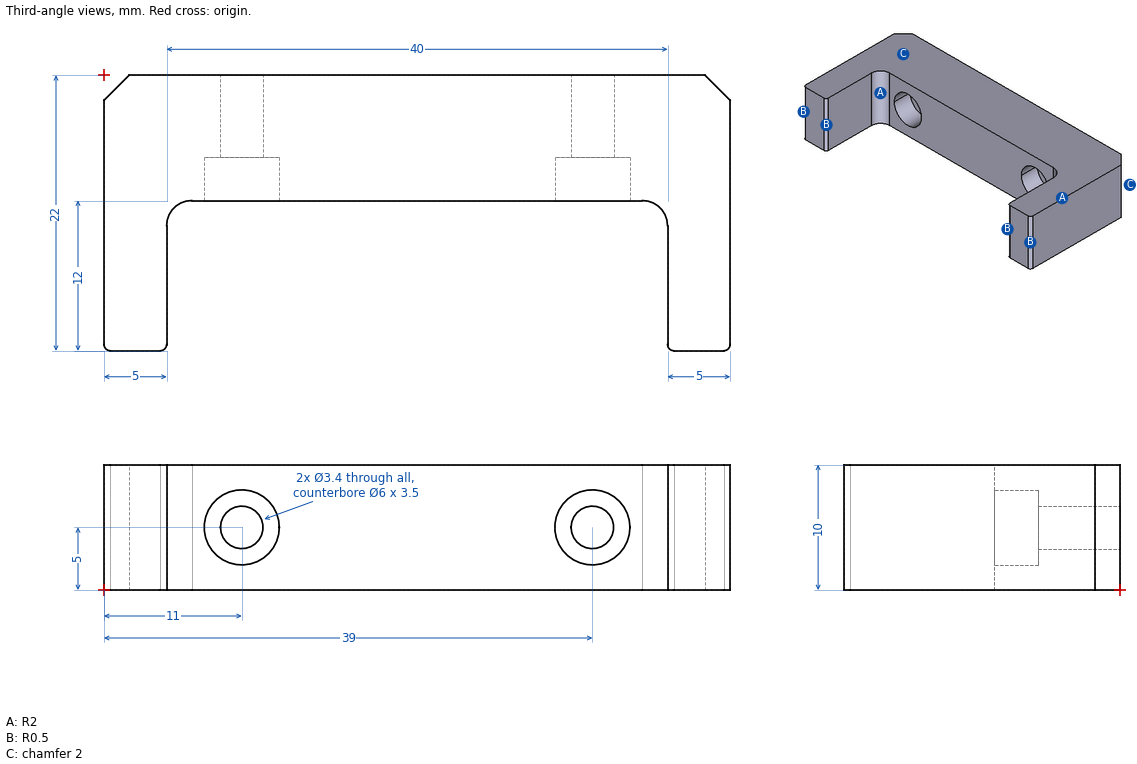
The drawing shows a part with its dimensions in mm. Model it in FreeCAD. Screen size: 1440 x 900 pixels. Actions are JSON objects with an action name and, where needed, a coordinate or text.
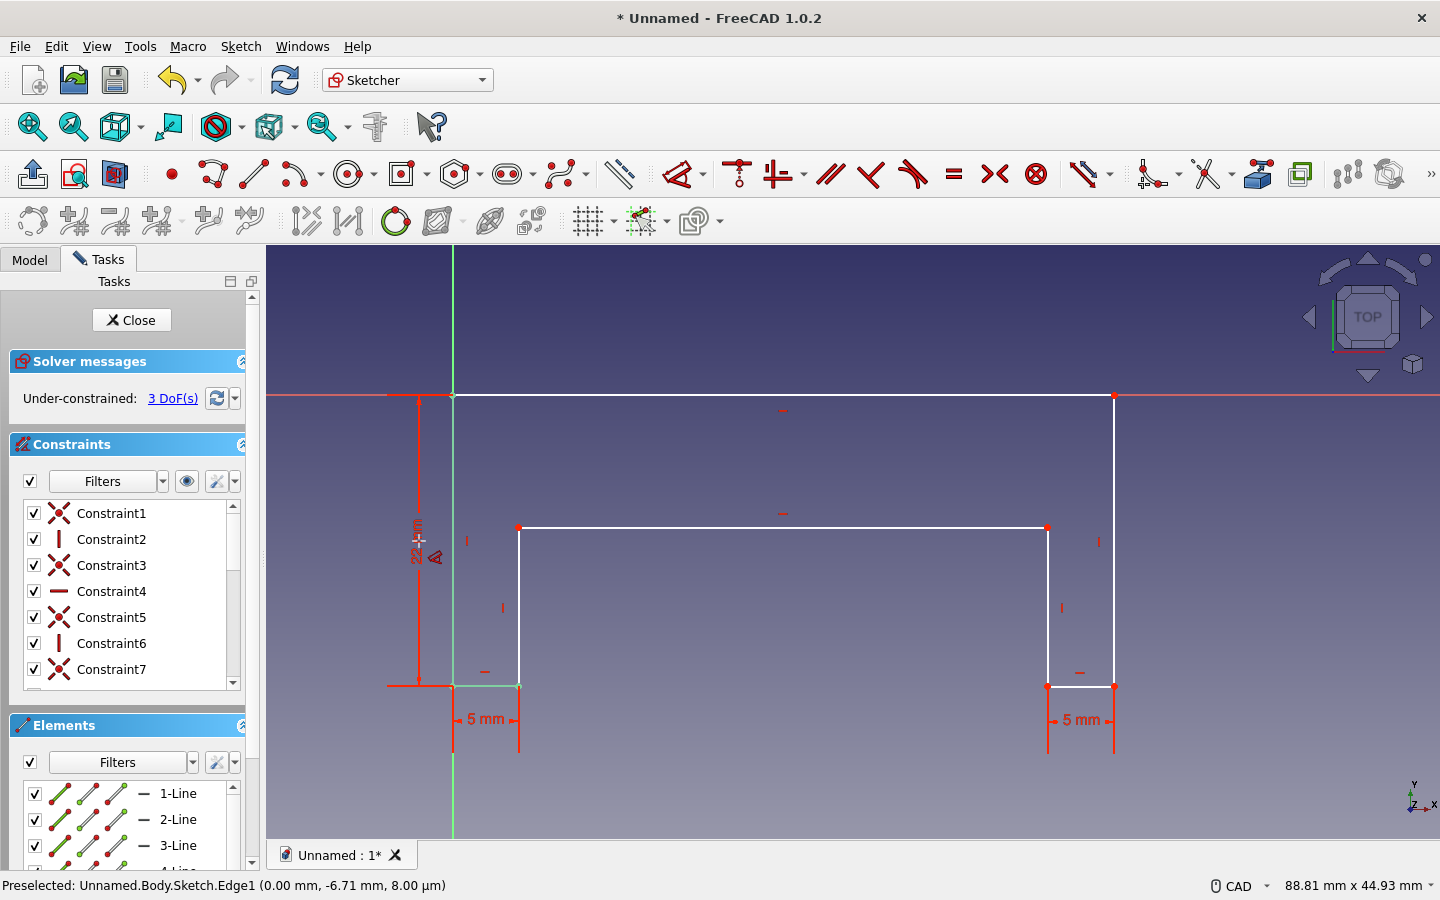
{"action": "left_click", "coordinate": [519, 639]}
{"action": "left_click", "coordinate": [485, 607]}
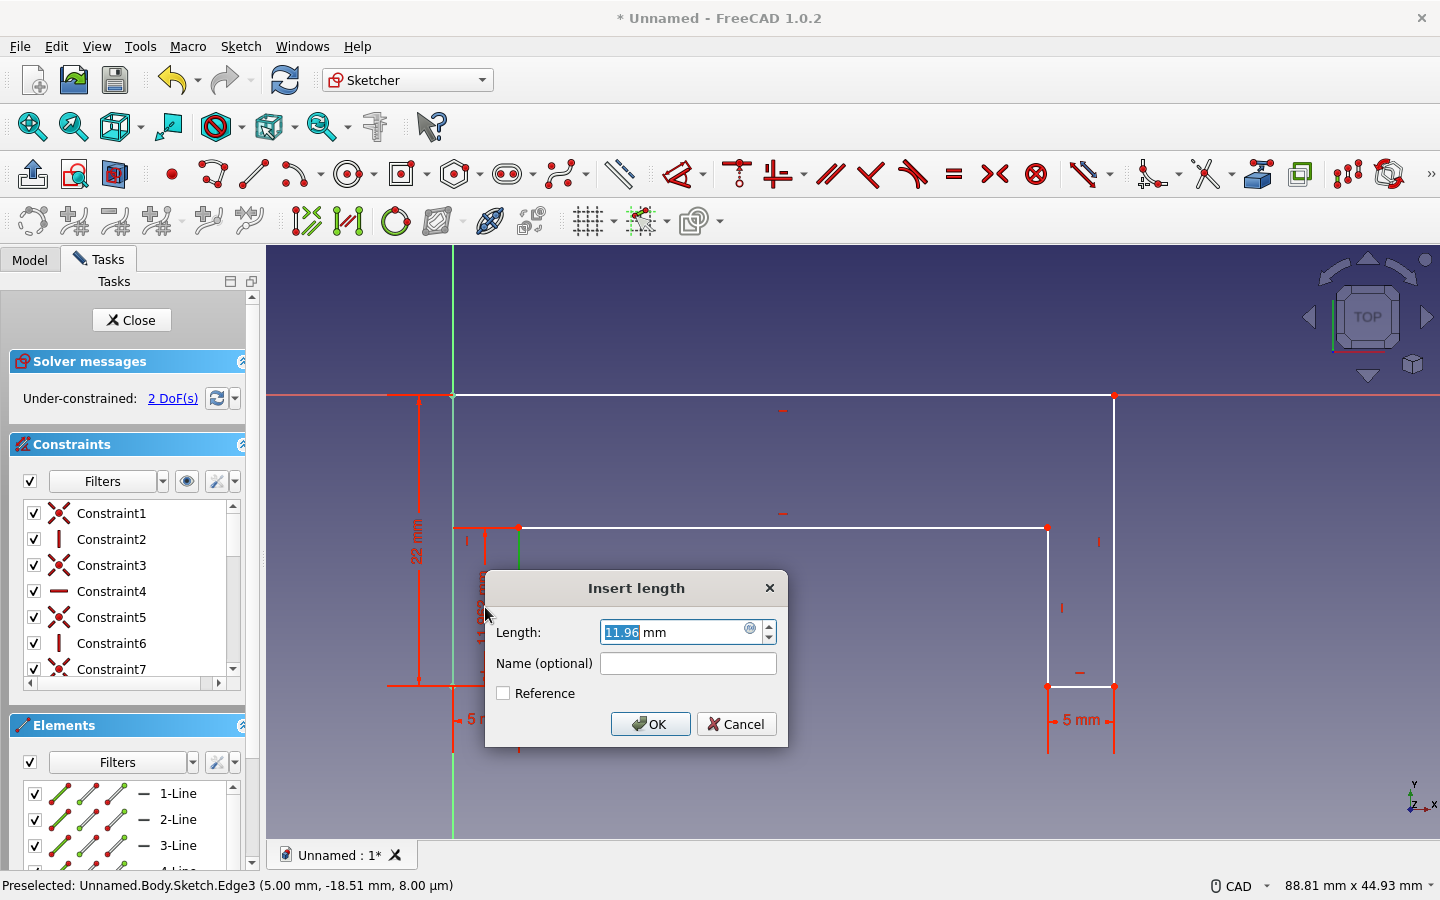
{"action": "type", "text": "12"}
{"action": "key", "text": "Return"}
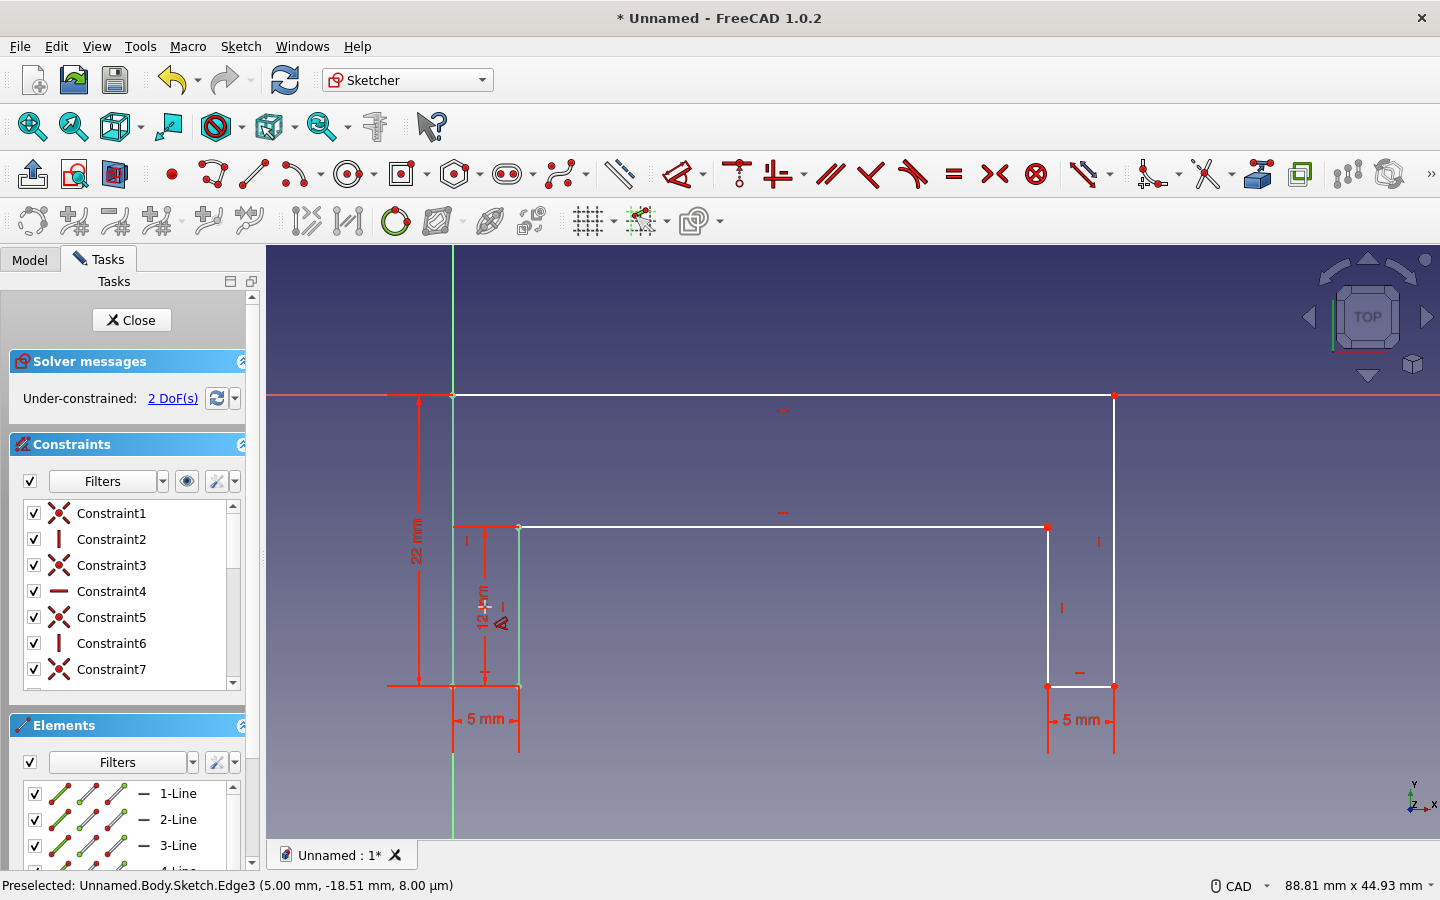
{"action": "left_click", "coordinate": [677, 527]}
{"action": "left_click", "coordinate": [783, 493]}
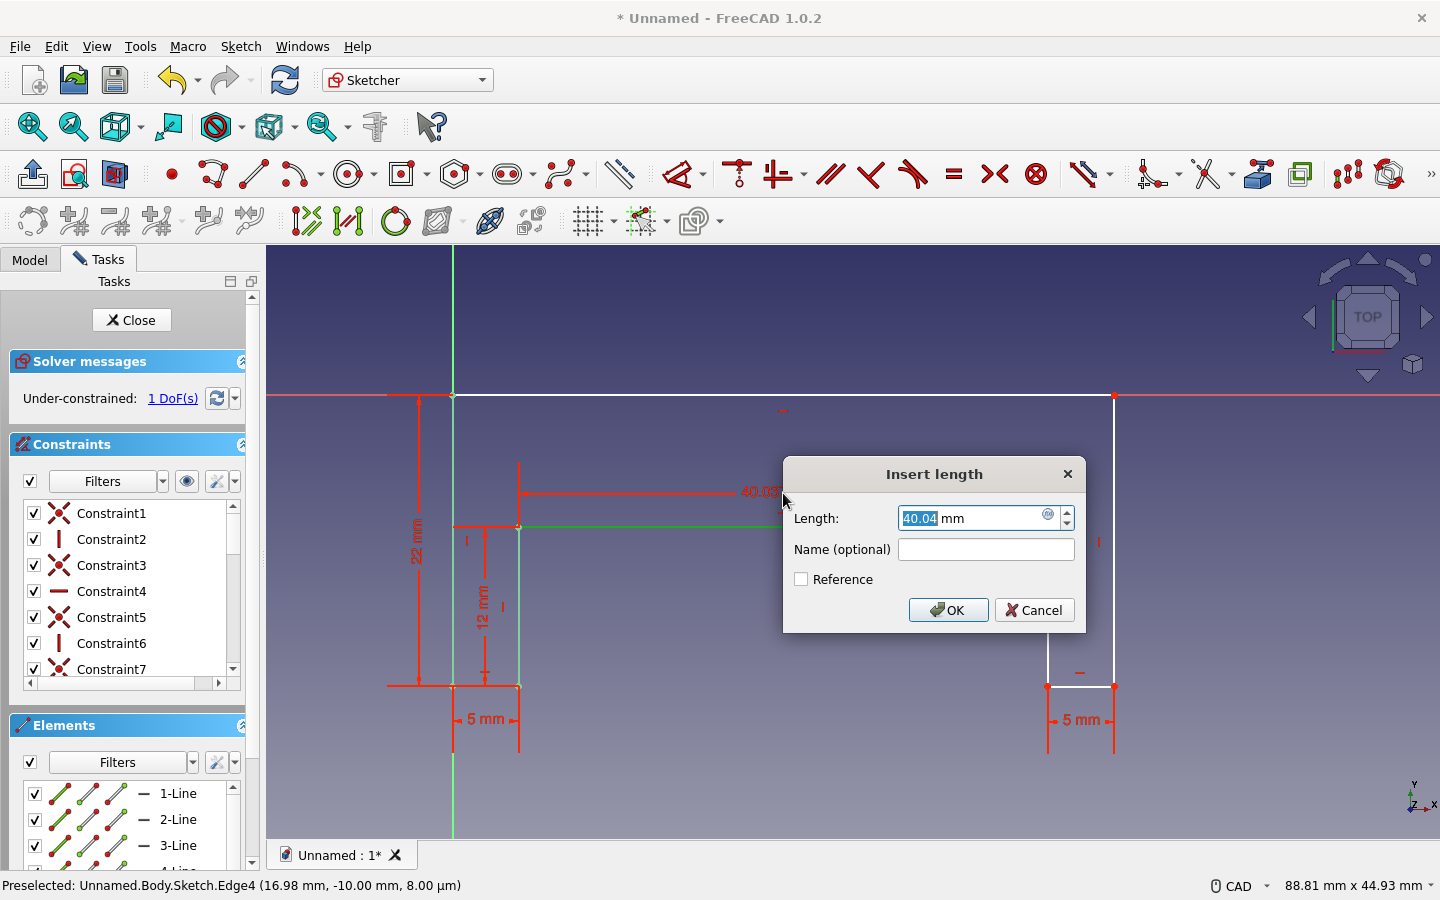
{"action": "type", "text": "40"}
{"action": "key", "text": "Return"}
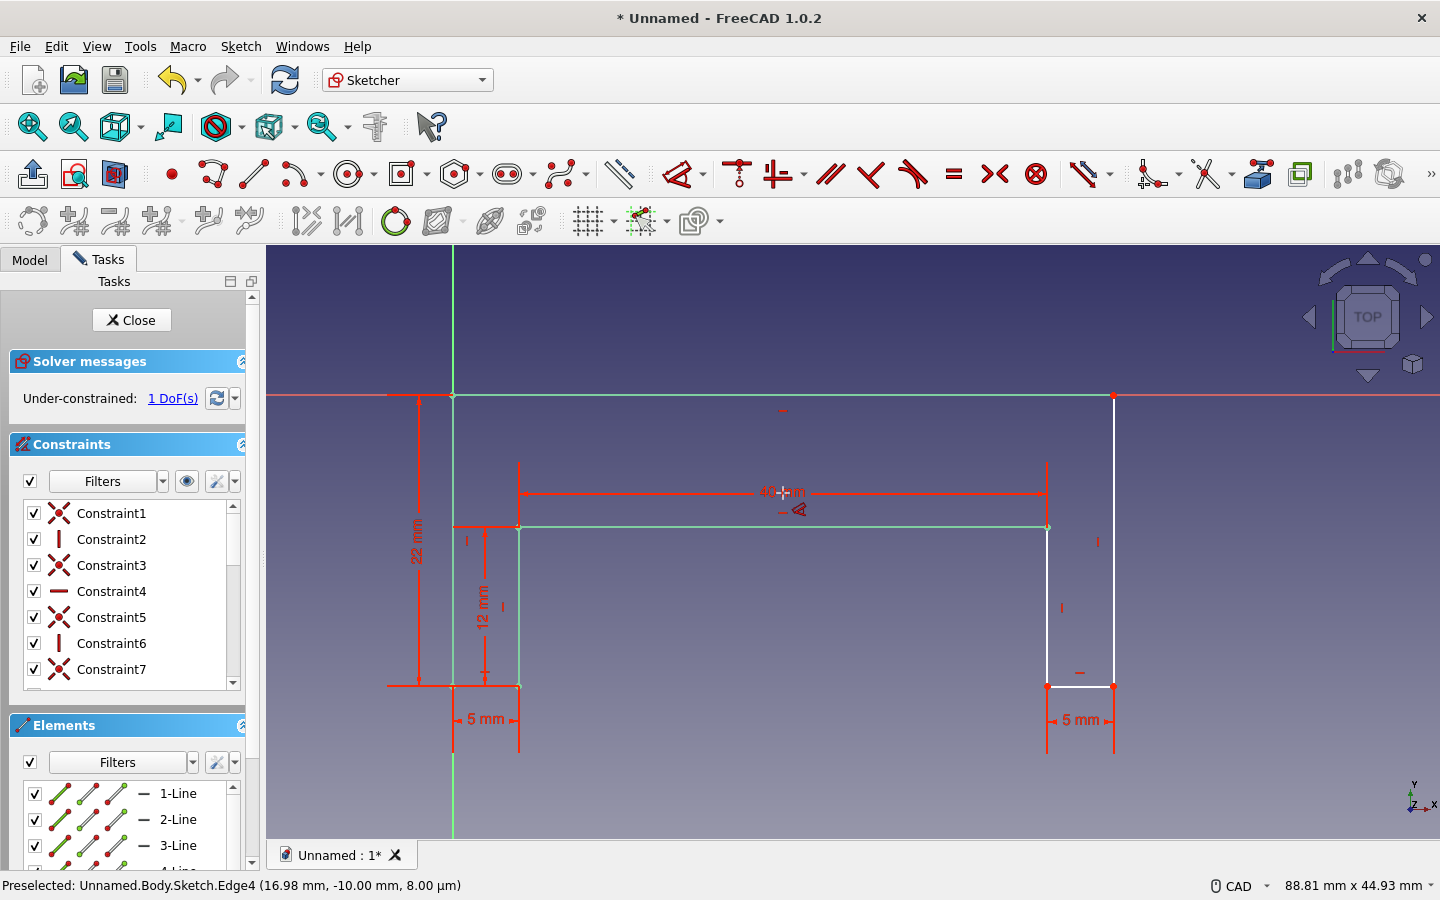
{"action": "left_click", "coordinate": [1047, 575]}
{"action": "left_click", "coordinate": [1081, 607]}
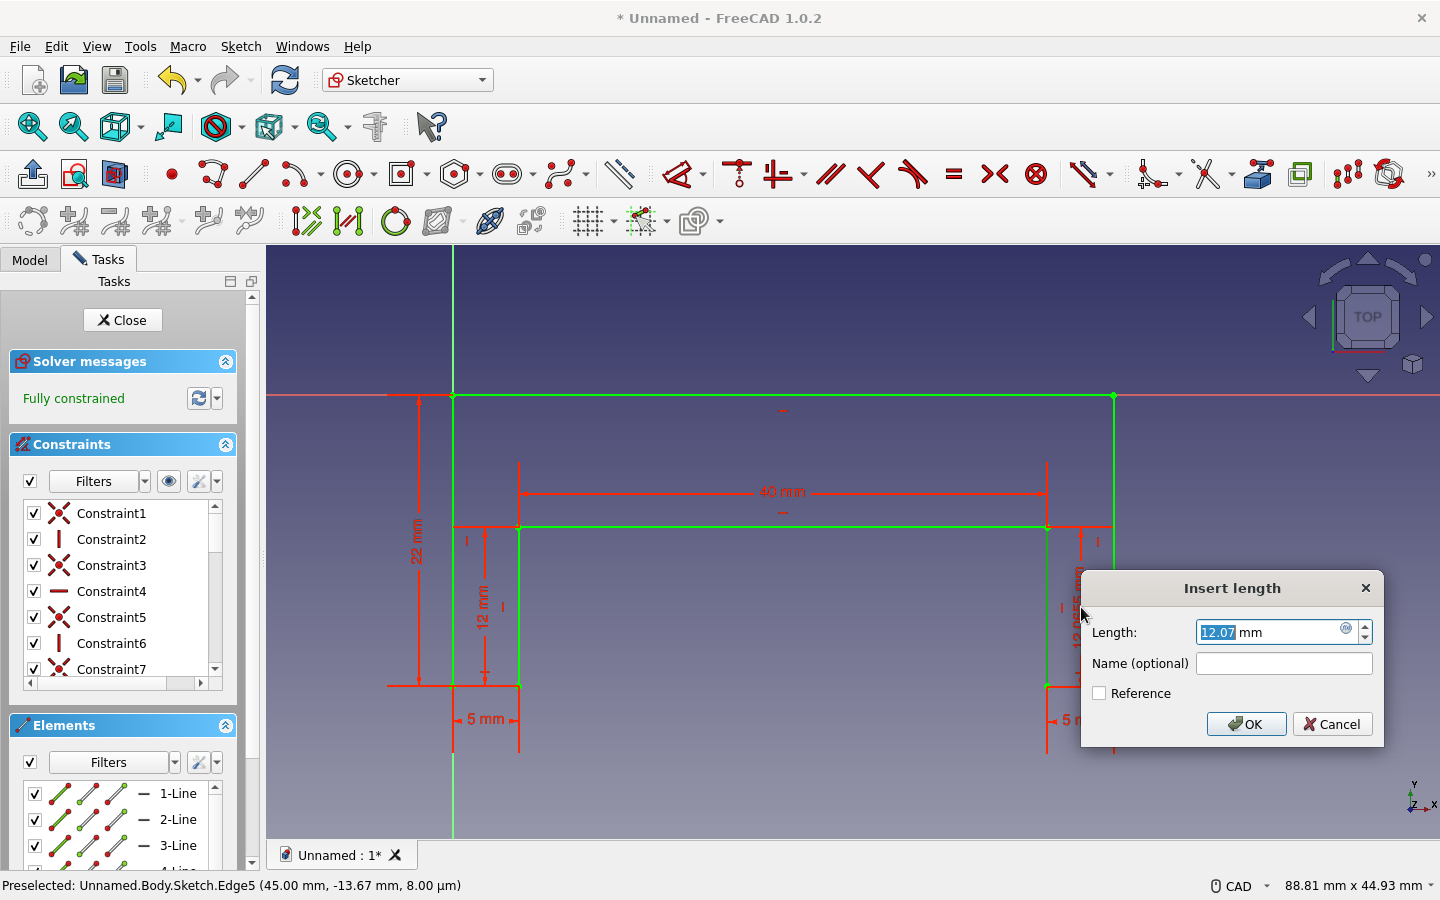
{"action": "type", "text": "12"}
{"action": "key", "text": "Return"}
{"action": "key", "text": "Escape"}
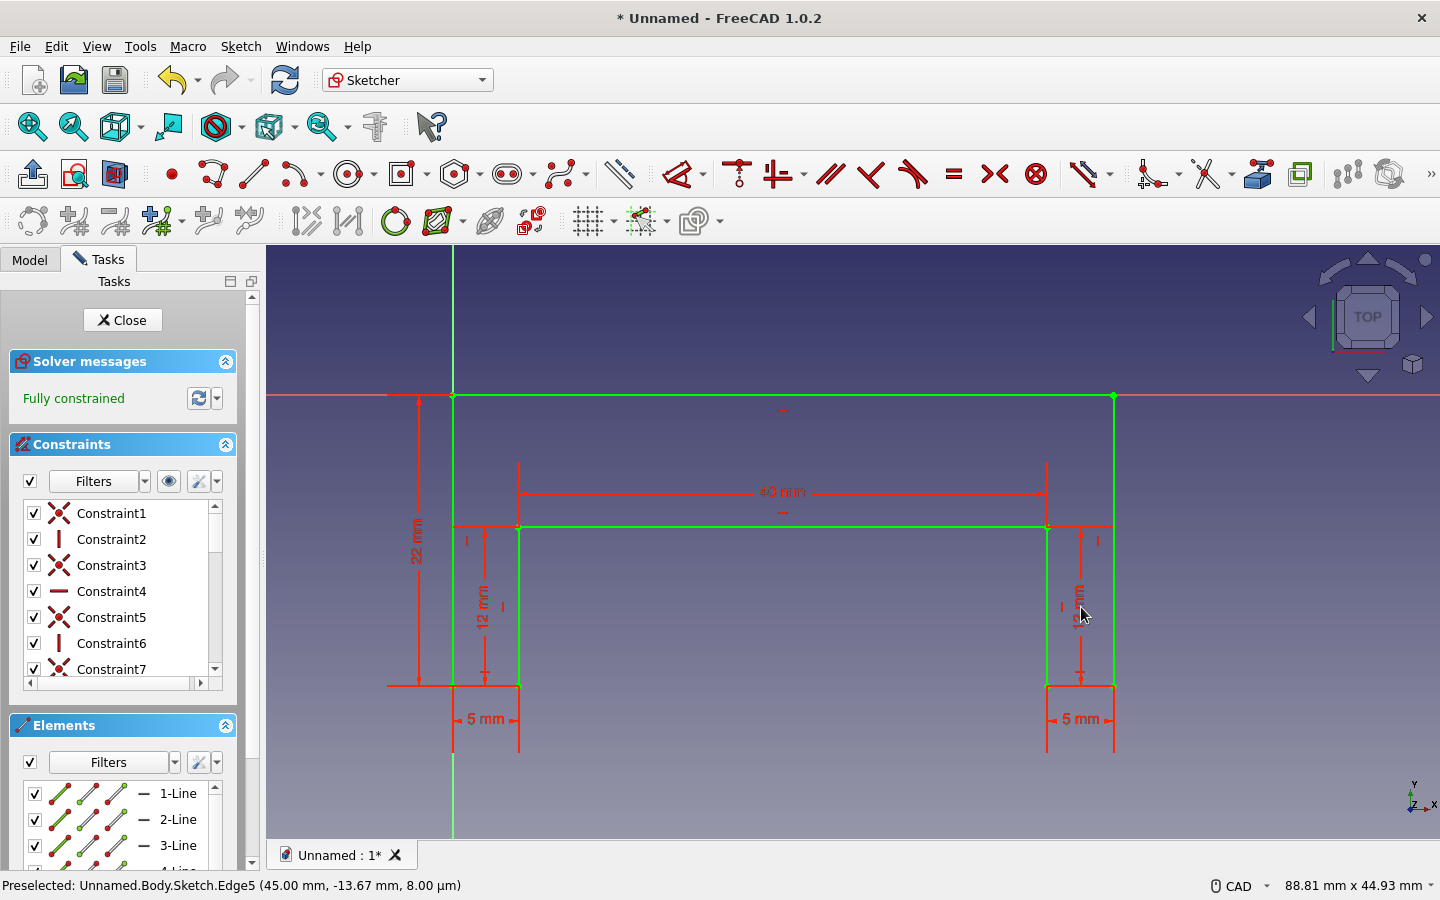
{"action": "left_click", "coordinate": [123, 320]}